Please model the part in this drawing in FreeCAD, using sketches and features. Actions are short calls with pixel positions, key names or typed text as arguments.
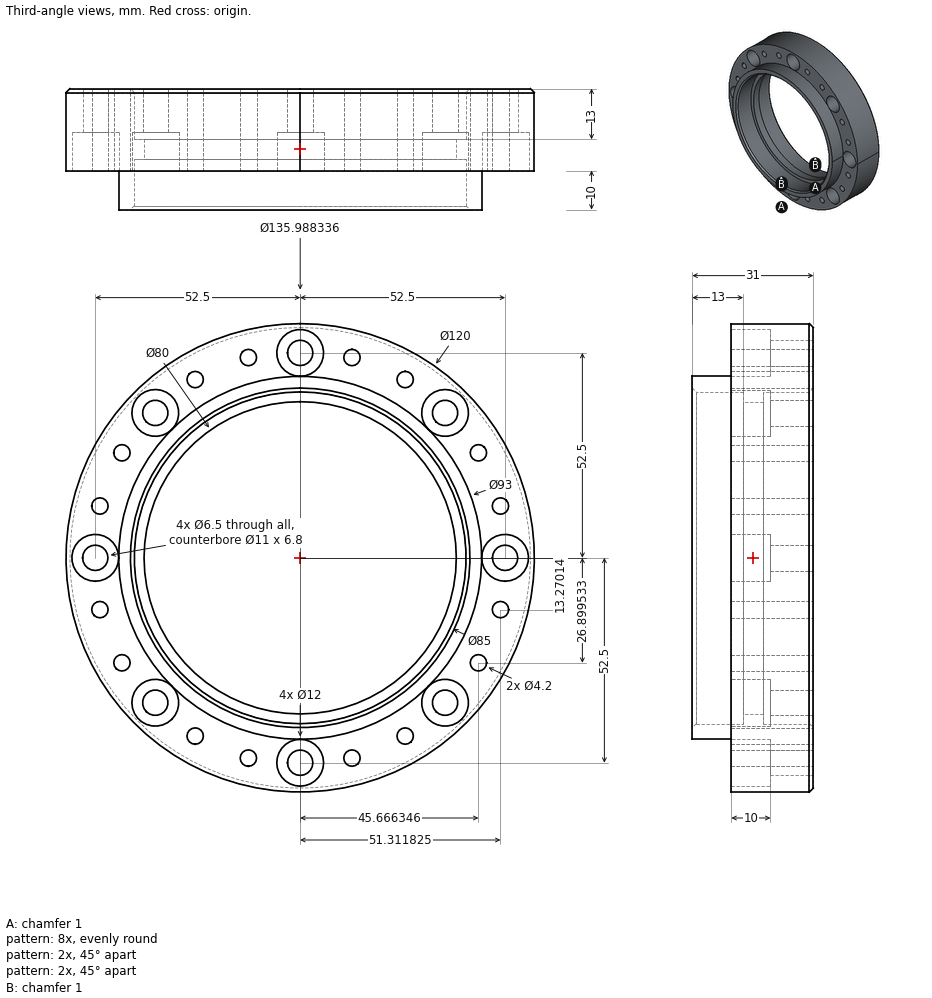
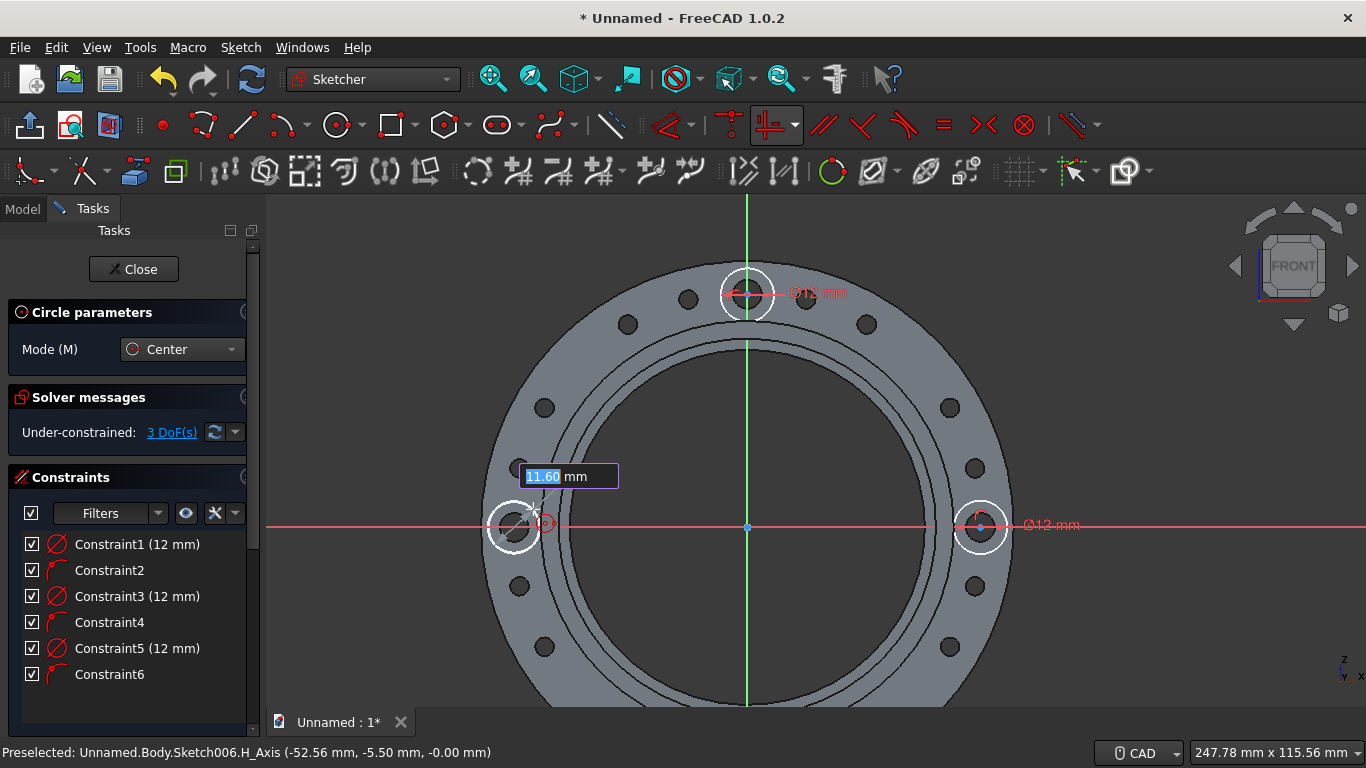
text(12)
key(Return)
key(Escape)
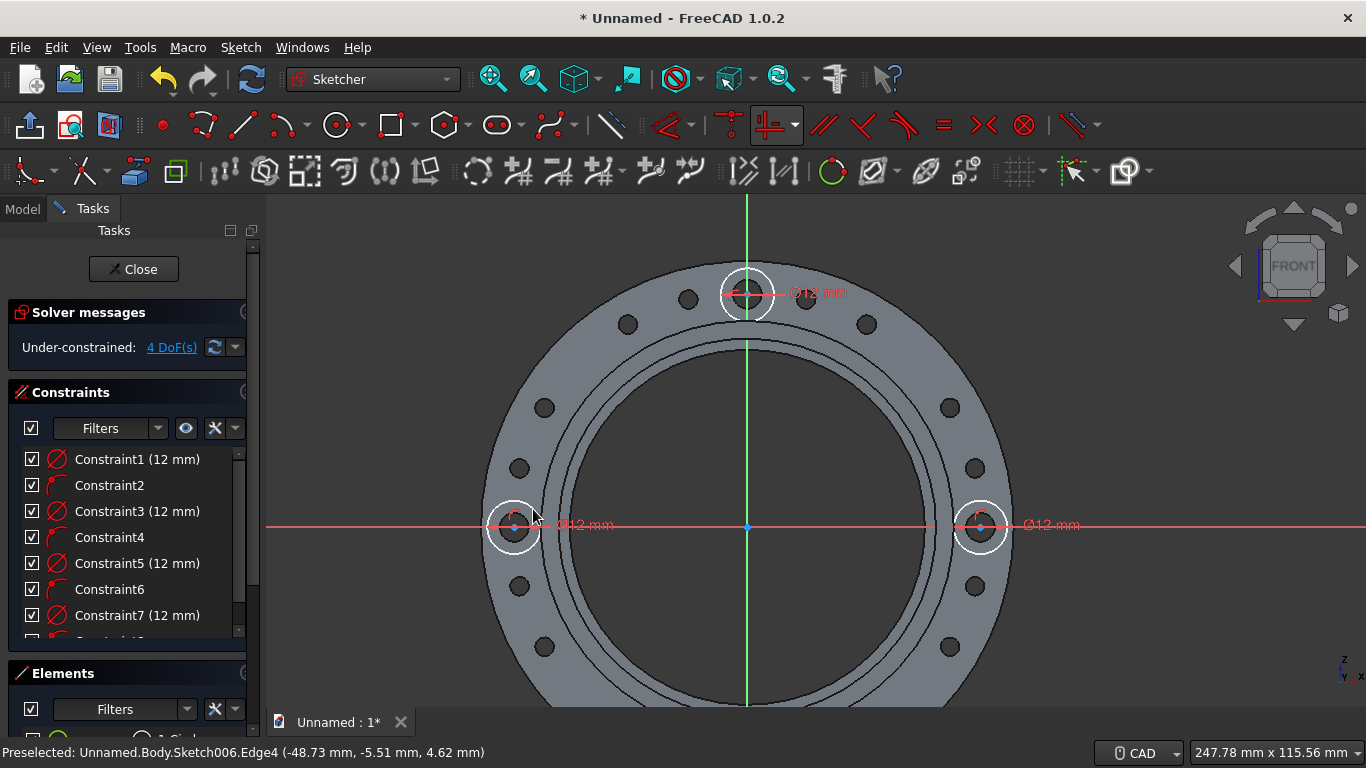
click(666, 126)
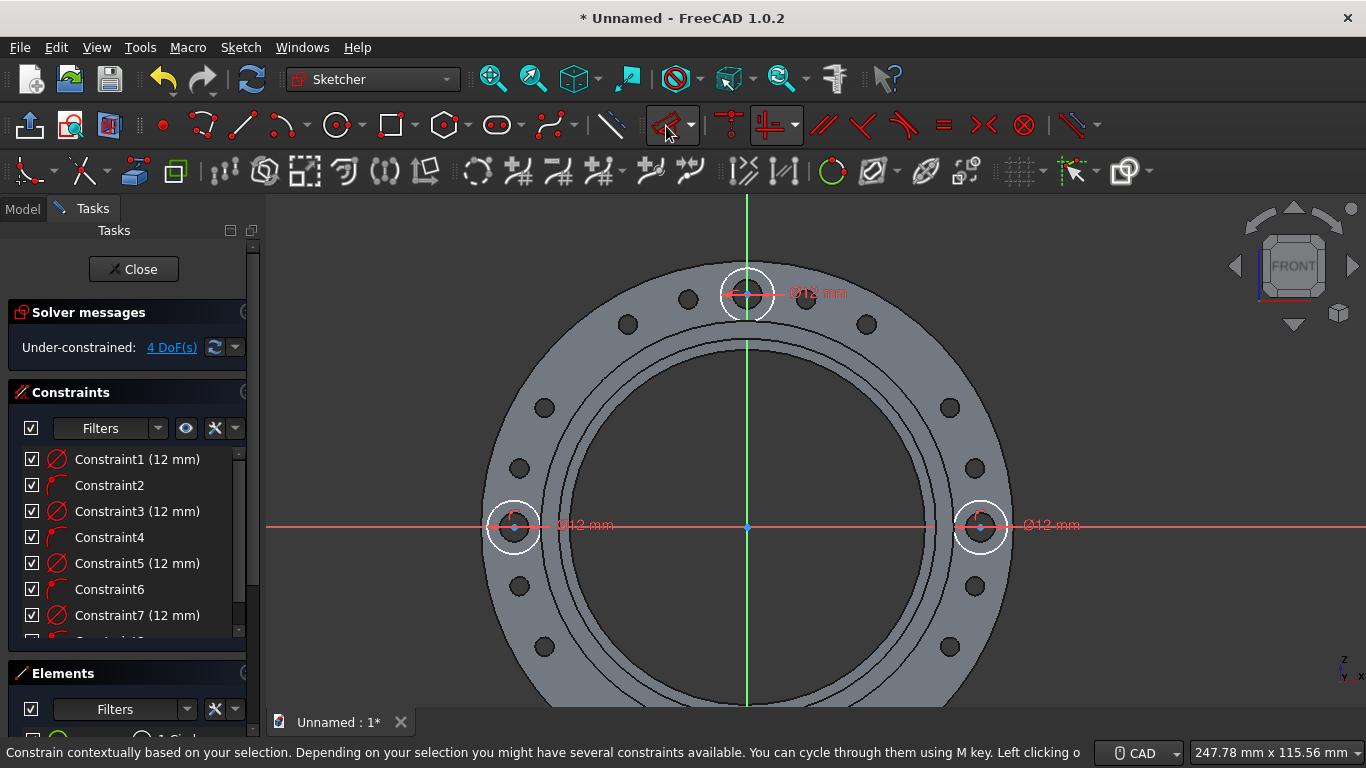
scroll(748, 294, down, 2)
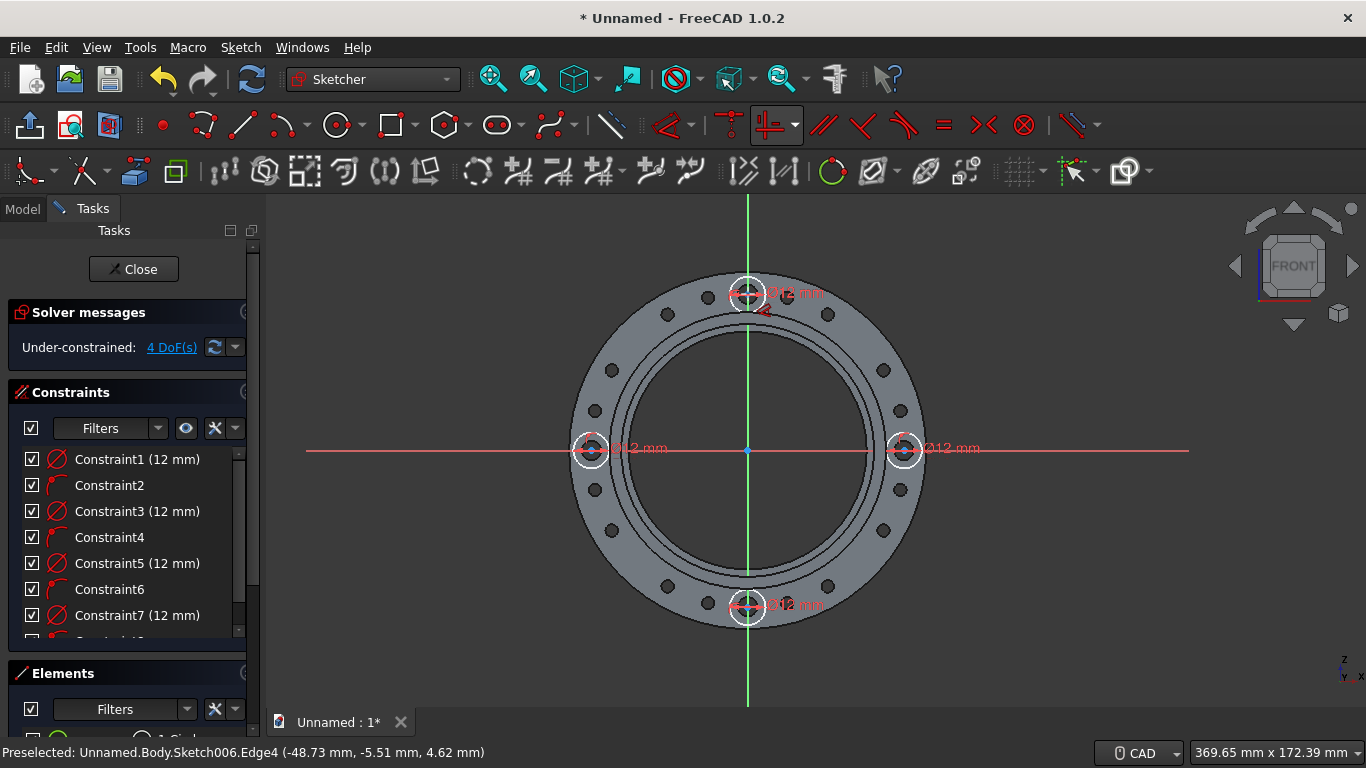
click(748, 607)
click(782, 529)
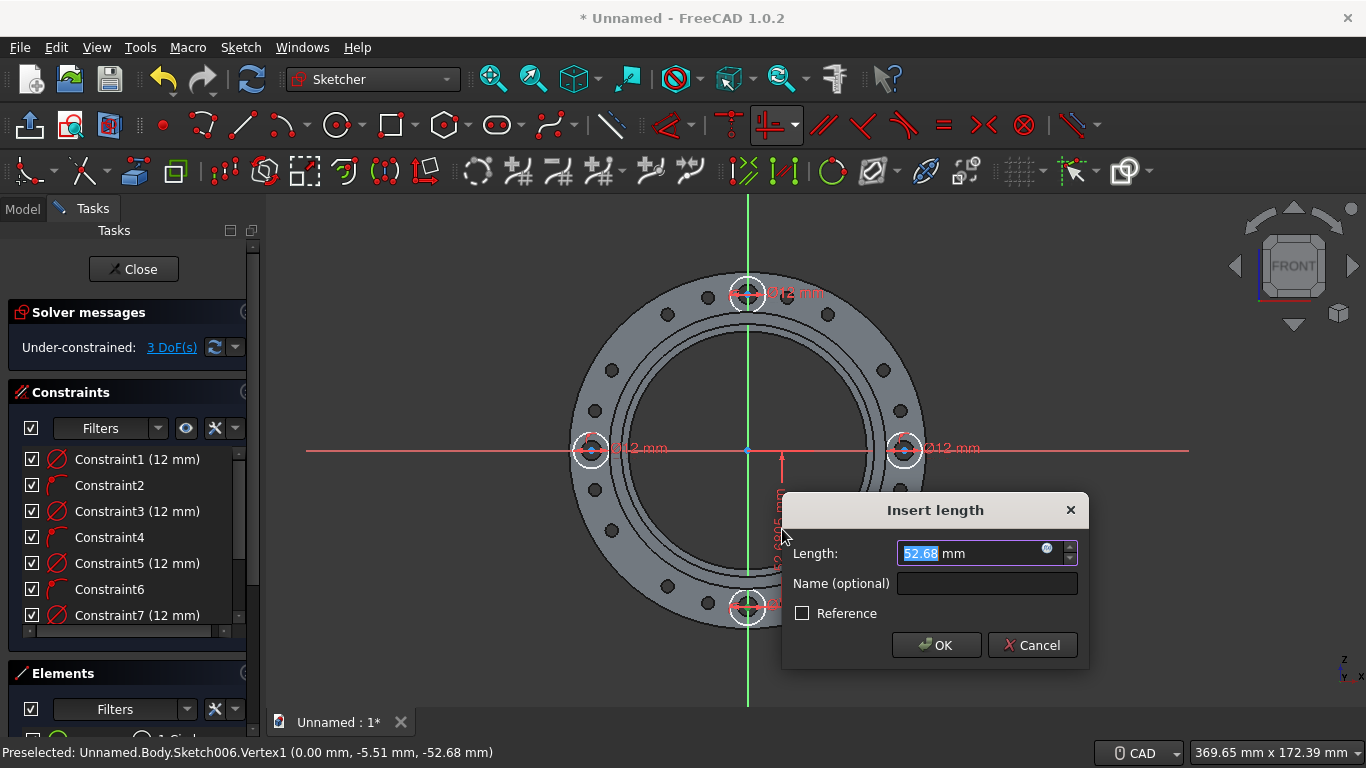
text(52.5)
key(Return)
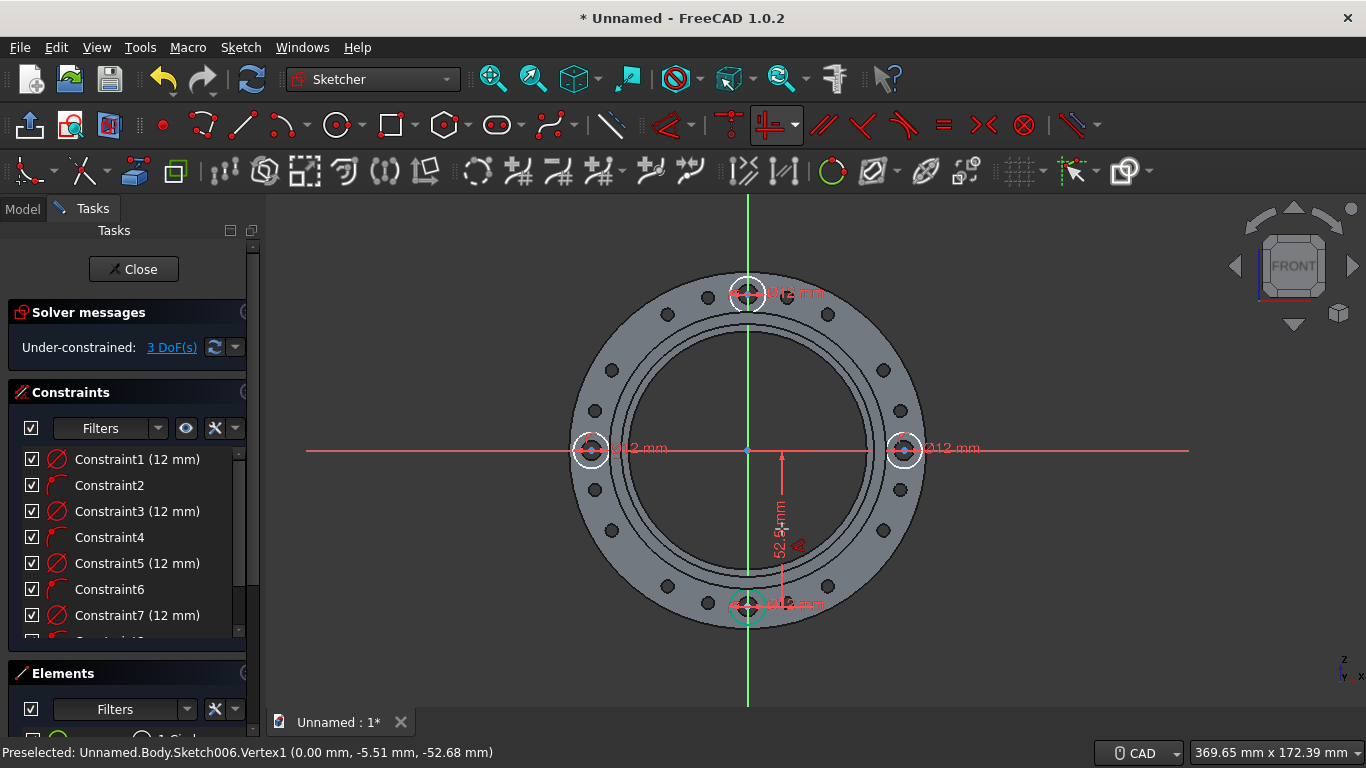
click(904, 450)
click(826, 484)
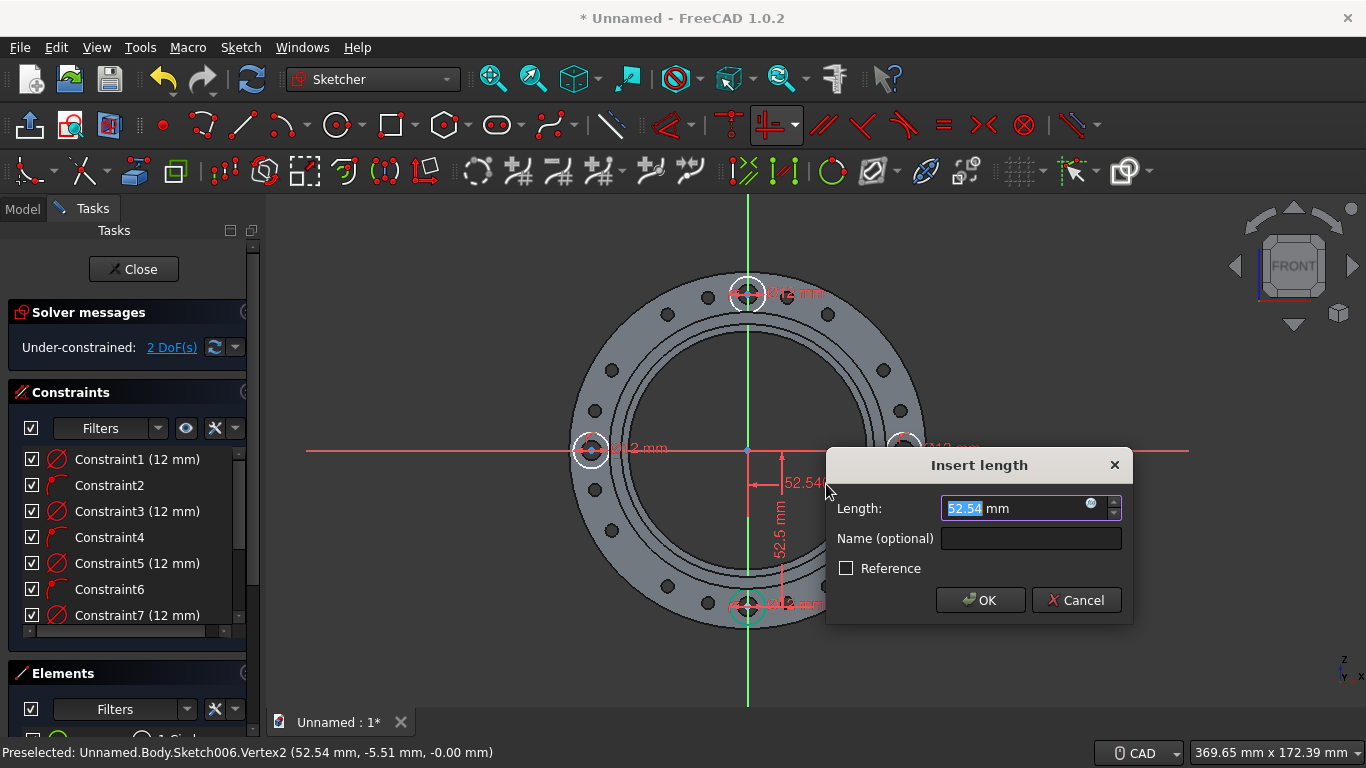
text(52.5)
key(Return)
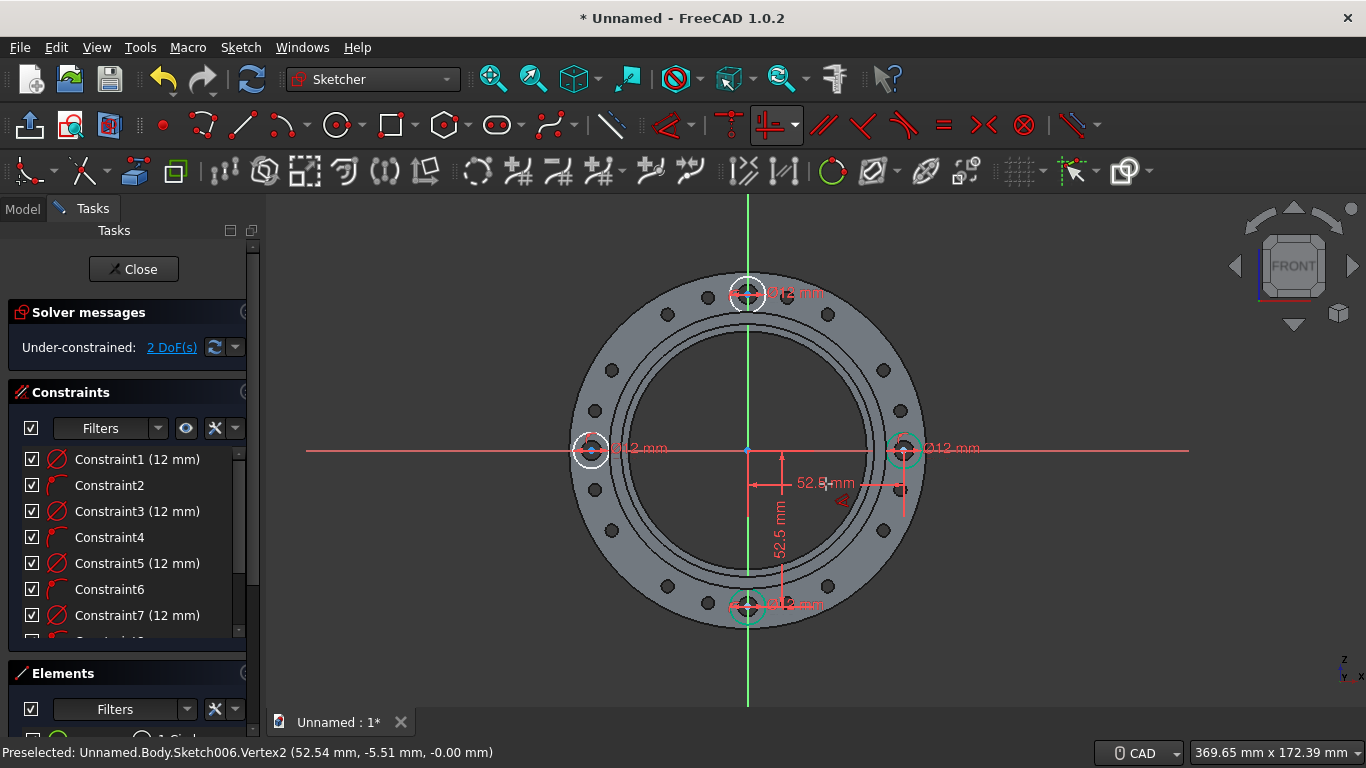
click(748, 295)
click(782, 373)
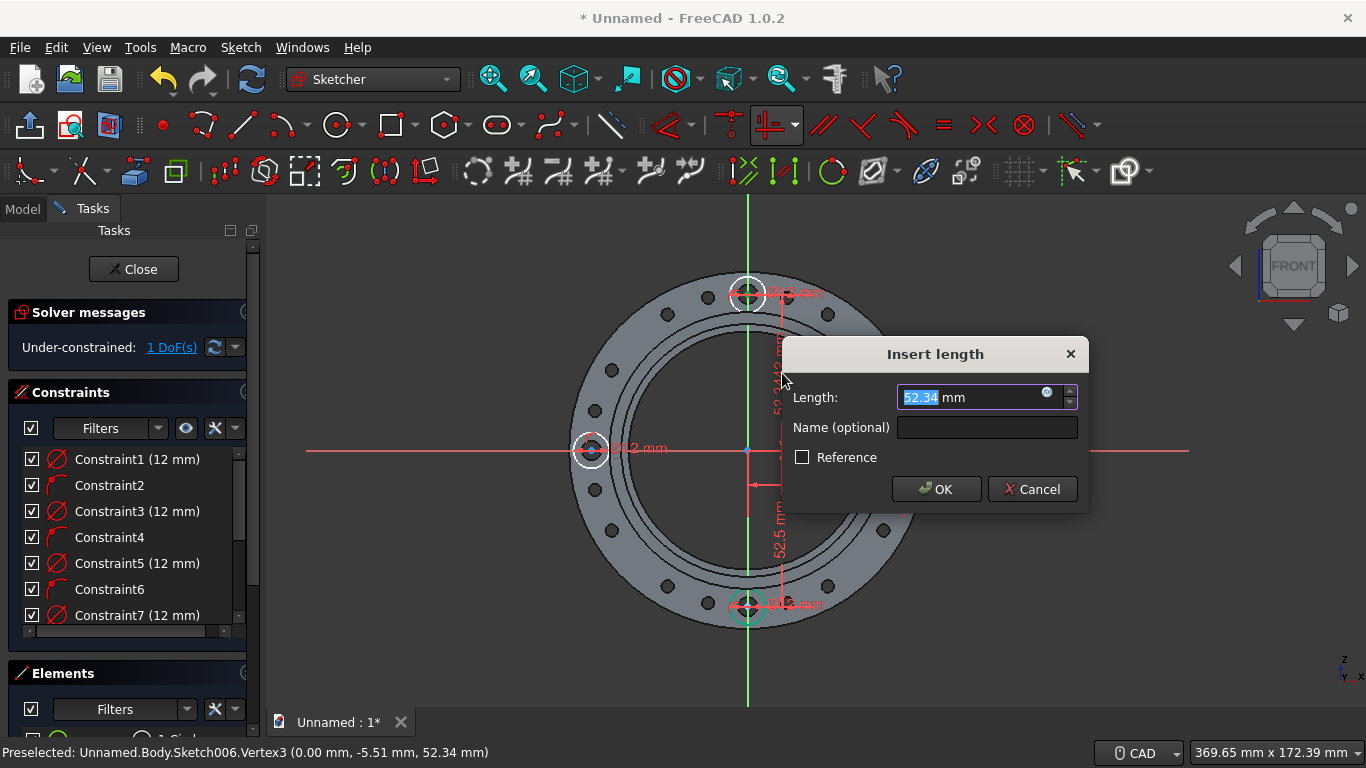
text(52.5)
key(Return)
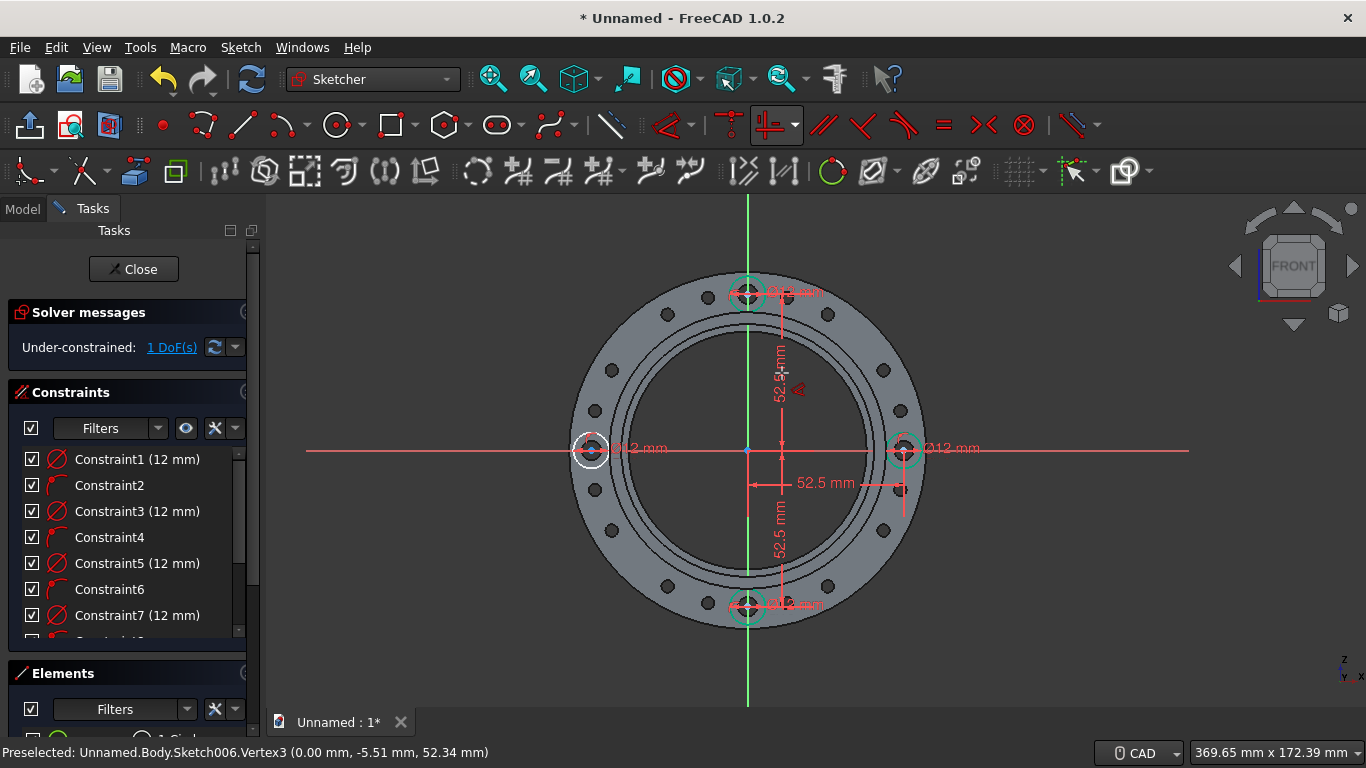
click(591, 450)
click(669, 484)